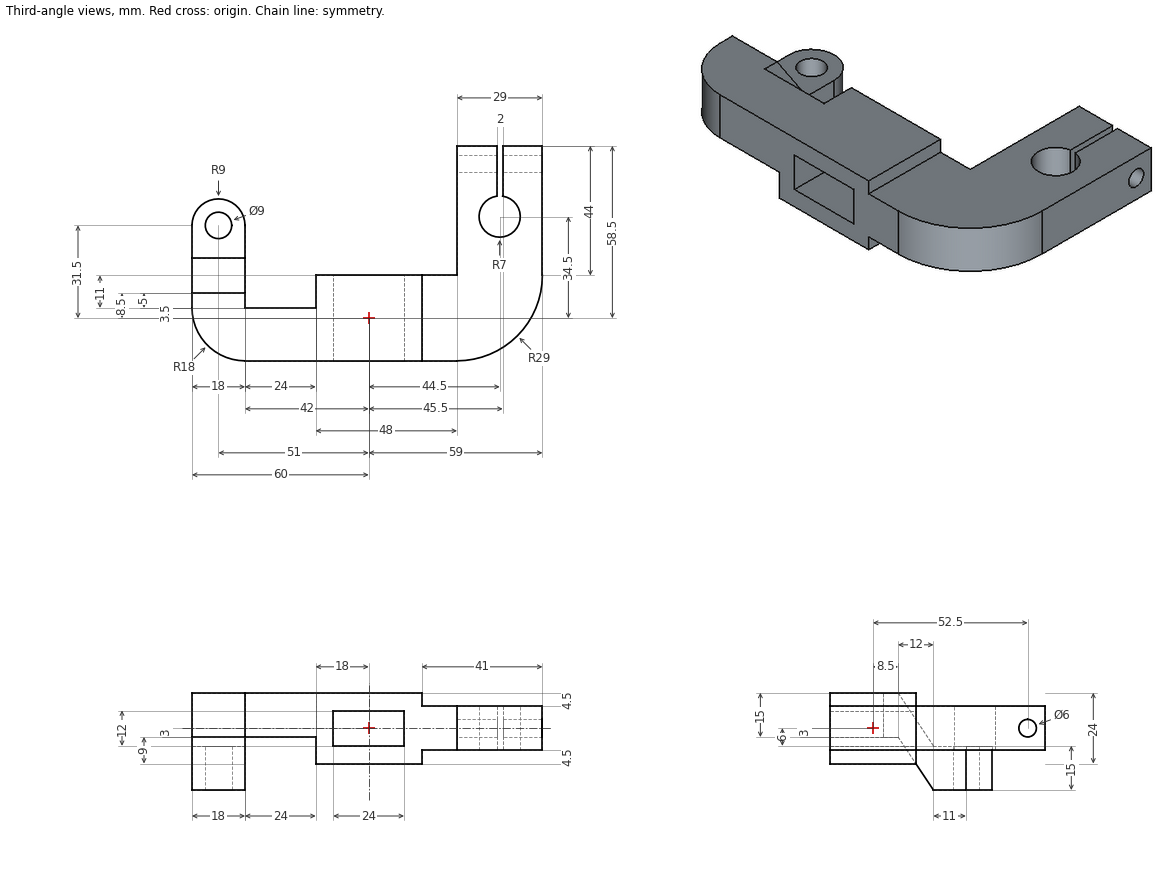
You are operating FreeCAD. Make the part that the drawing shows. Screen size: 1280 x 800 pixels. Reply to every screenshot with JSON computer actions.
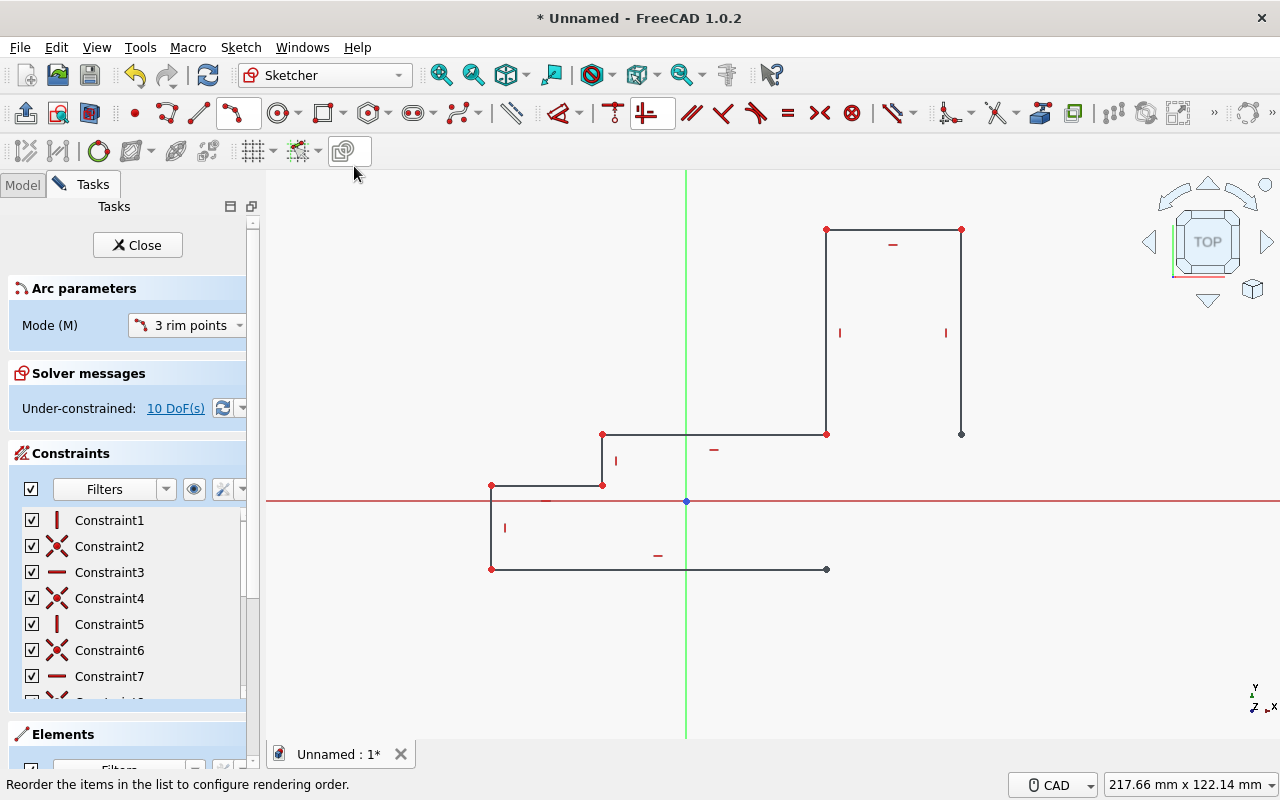
{"action": "left_click", "coordinate": [826, 570]}
{"action": "left_click", "coordinate": [961, 435]}
{"action": "left_click", "coordinate": [921, 529]}
{"action": "key", "text": "Escape"}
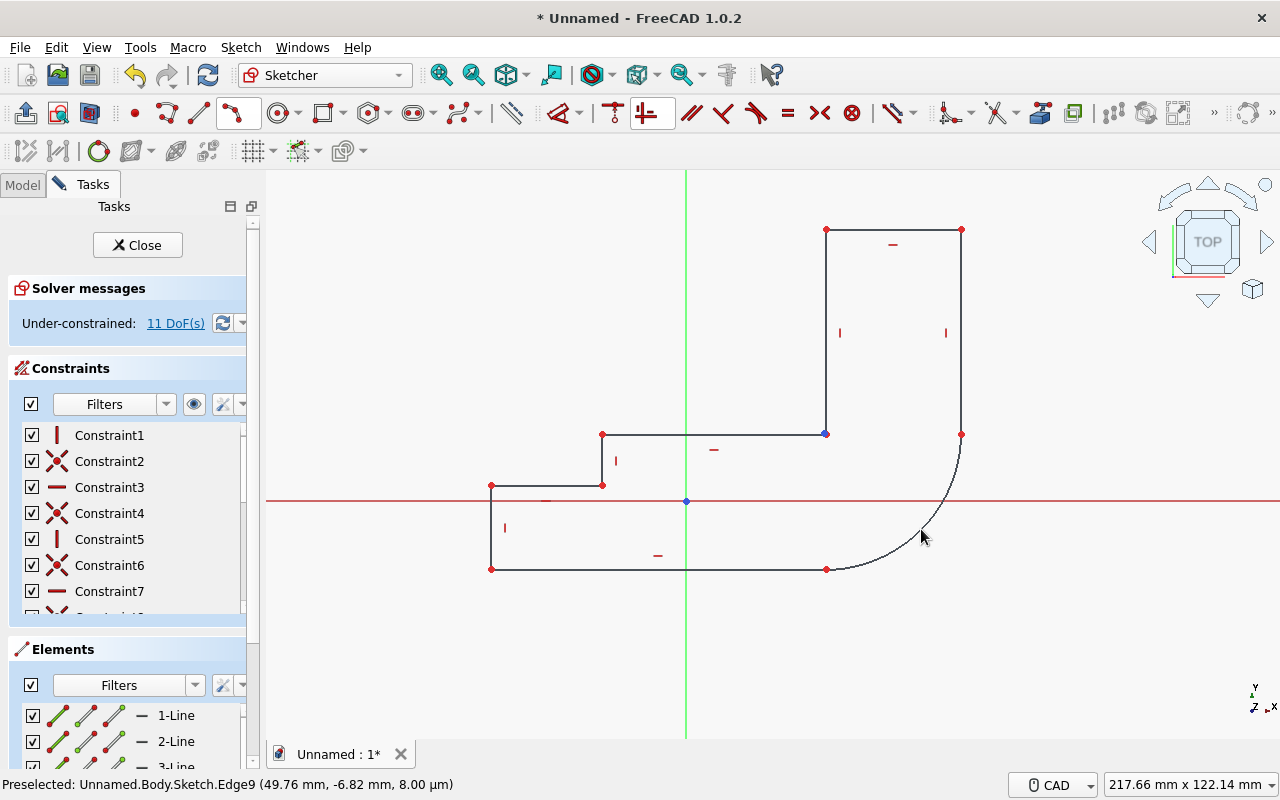
{"action": "left_click", "coordinate": [961, 373]}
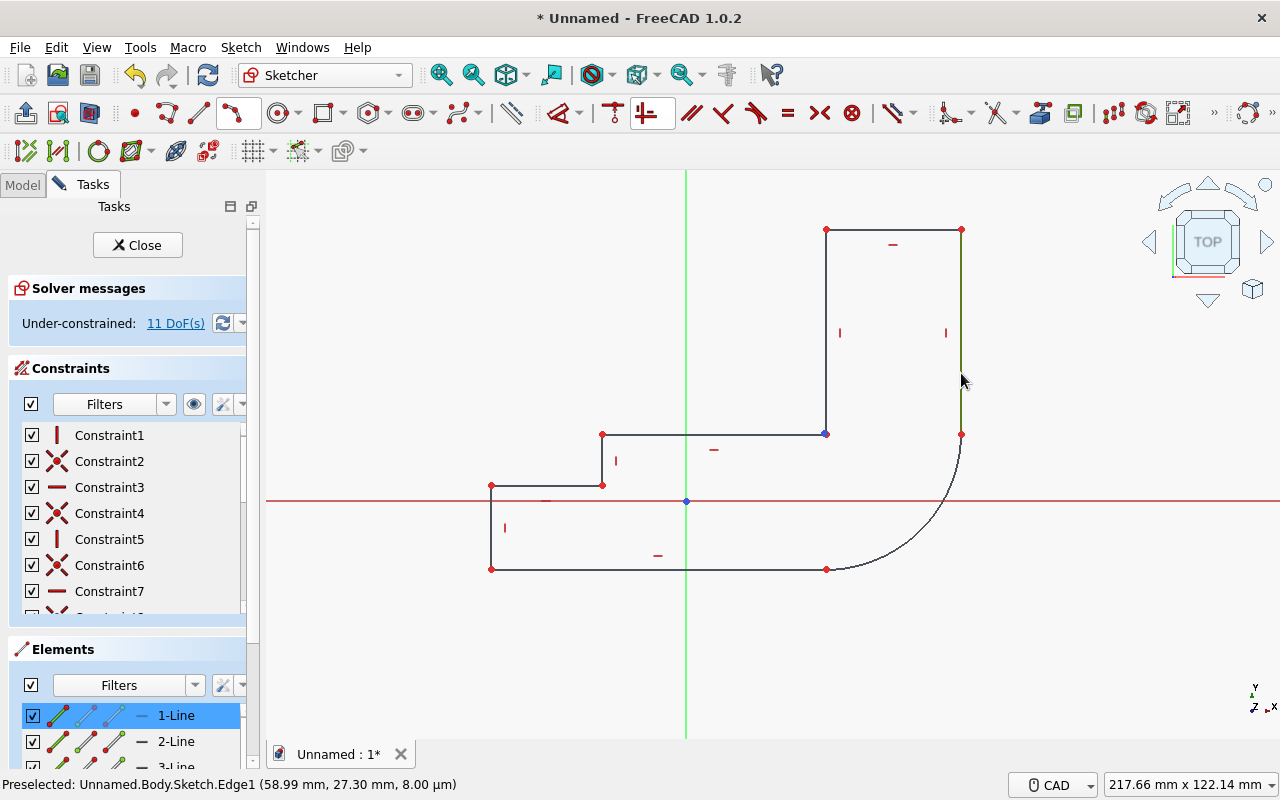
{"action": "left_click", "coordinate": [887, 555]}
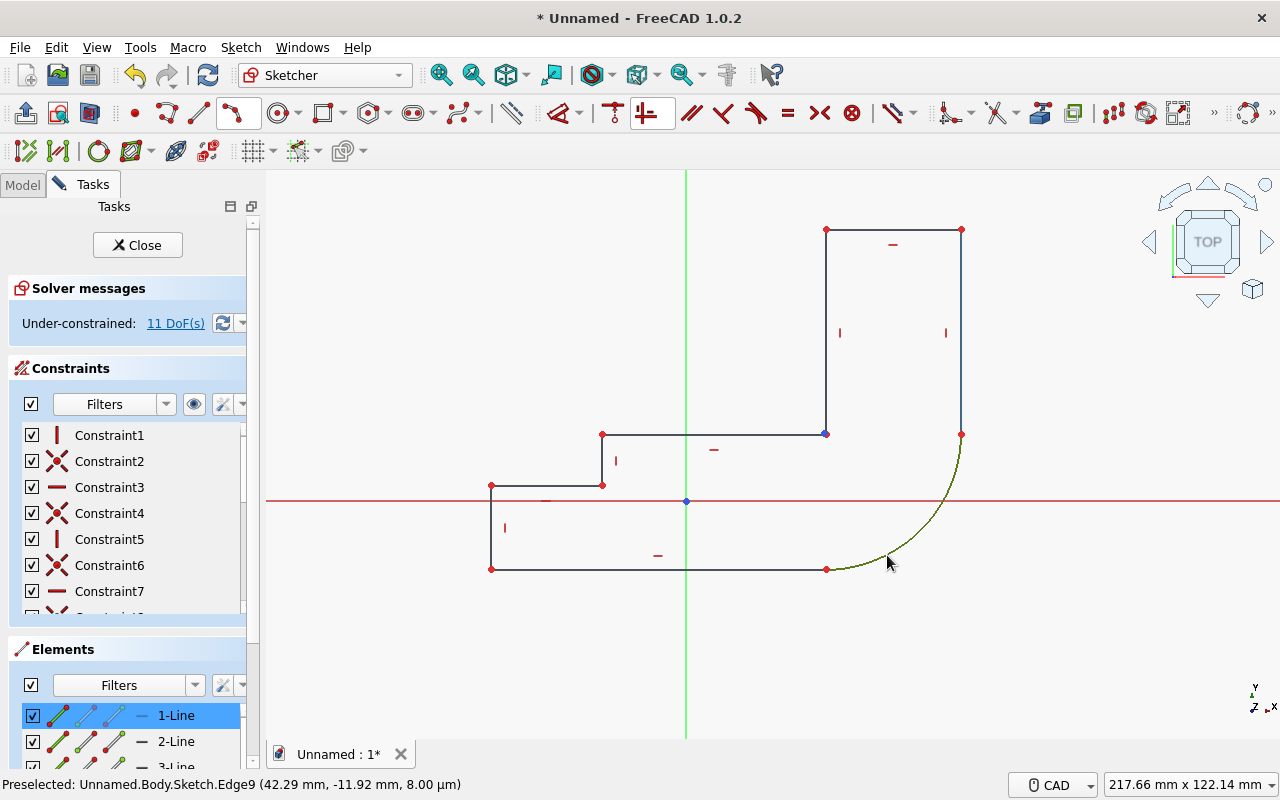
{"action": "left_click", "coordinate": [756, 114]}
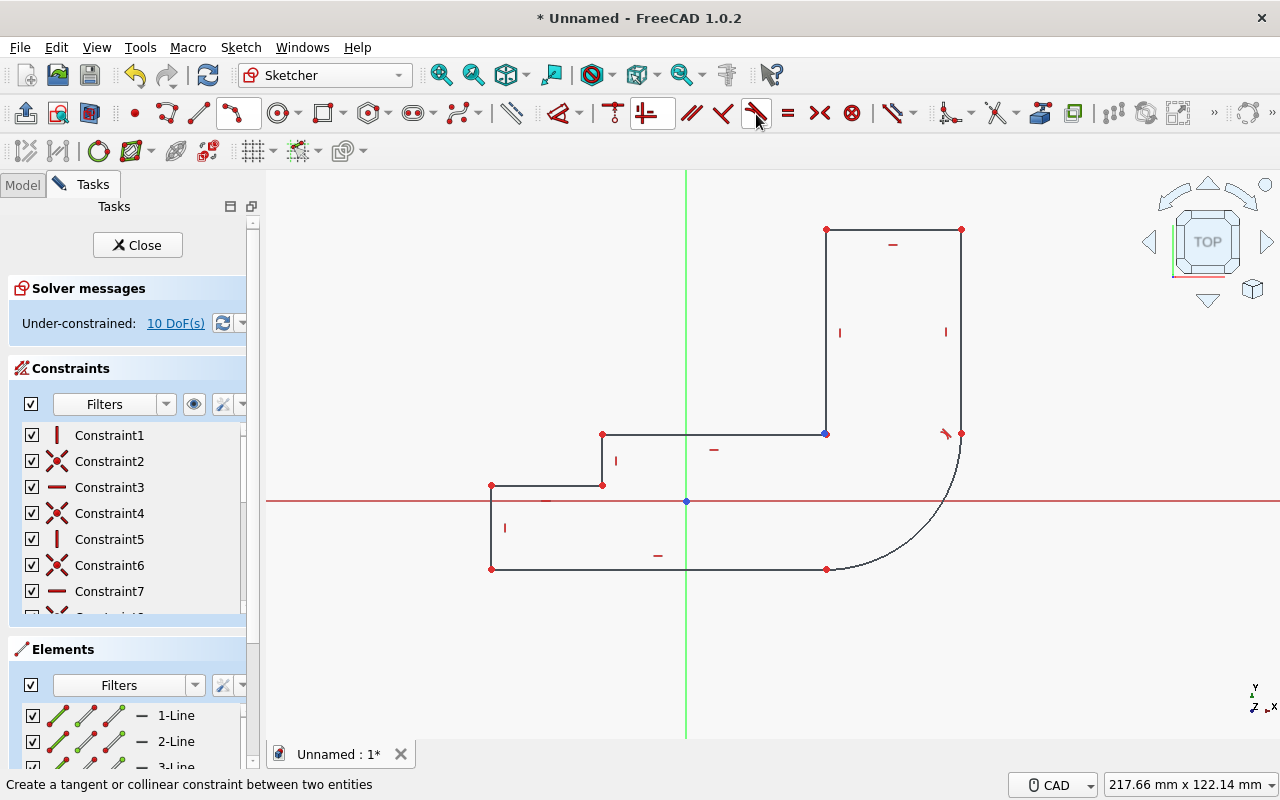
{"action": "left_click", "coordinate": [592, 570]}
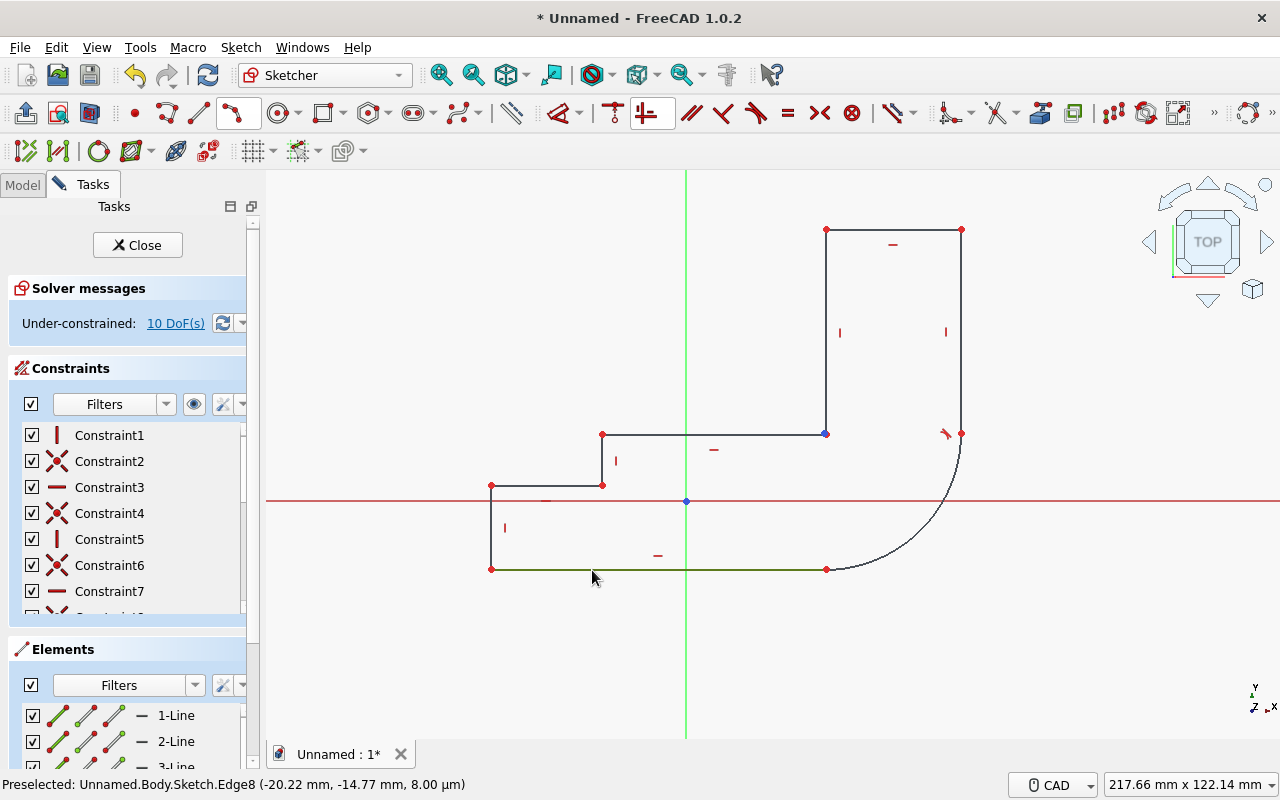
{"action": "left_click", "coordinate": [887, 555]}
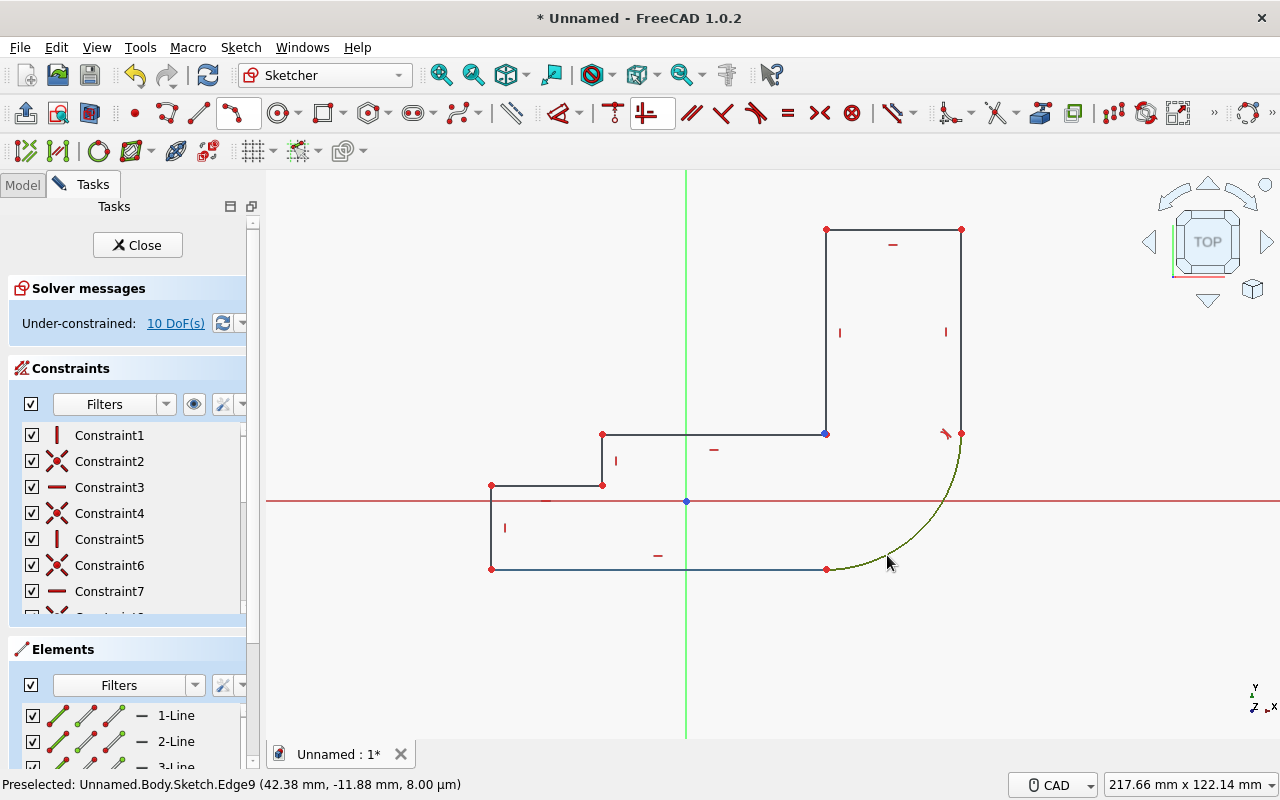
{"action": "left_click", "coordinate": [756, 114]}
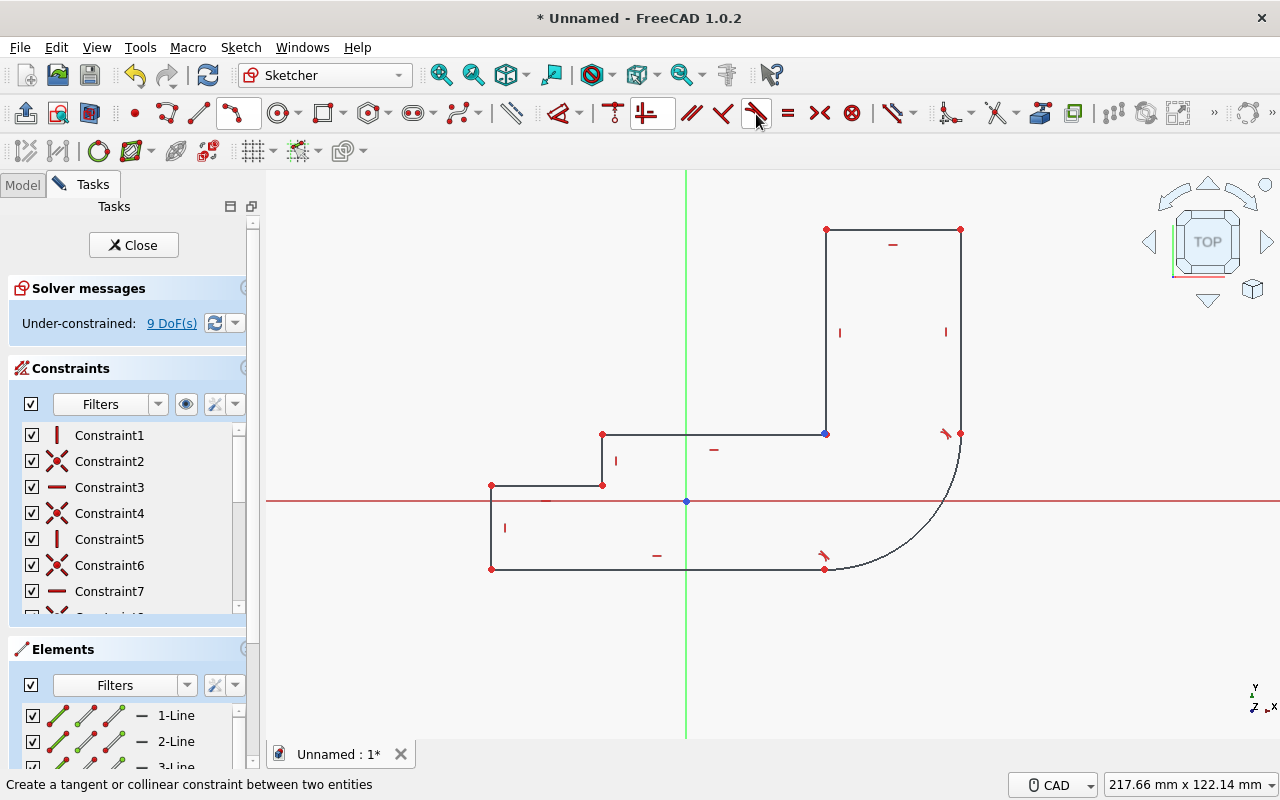
{"action": "left_click", "coordinate": [886, 555]}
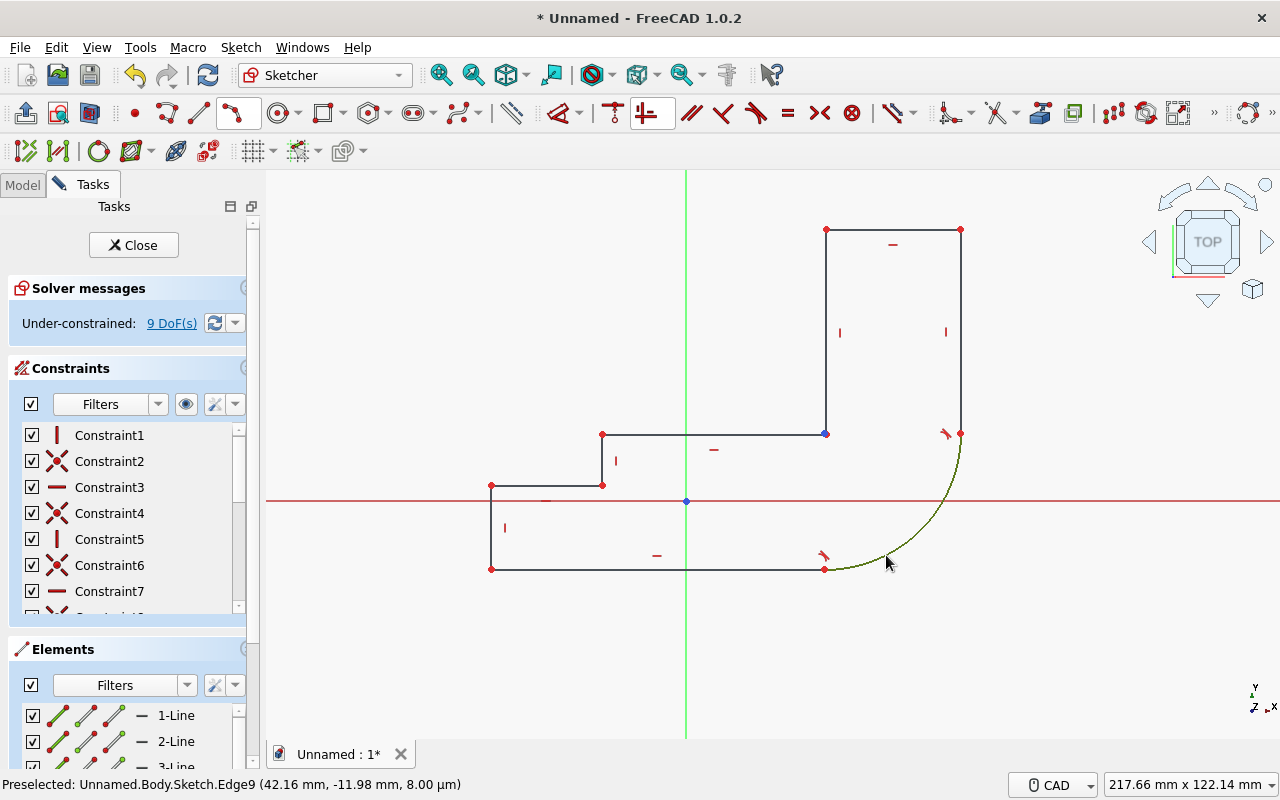
{"action": "left_click", "coordinate": [582, 114]}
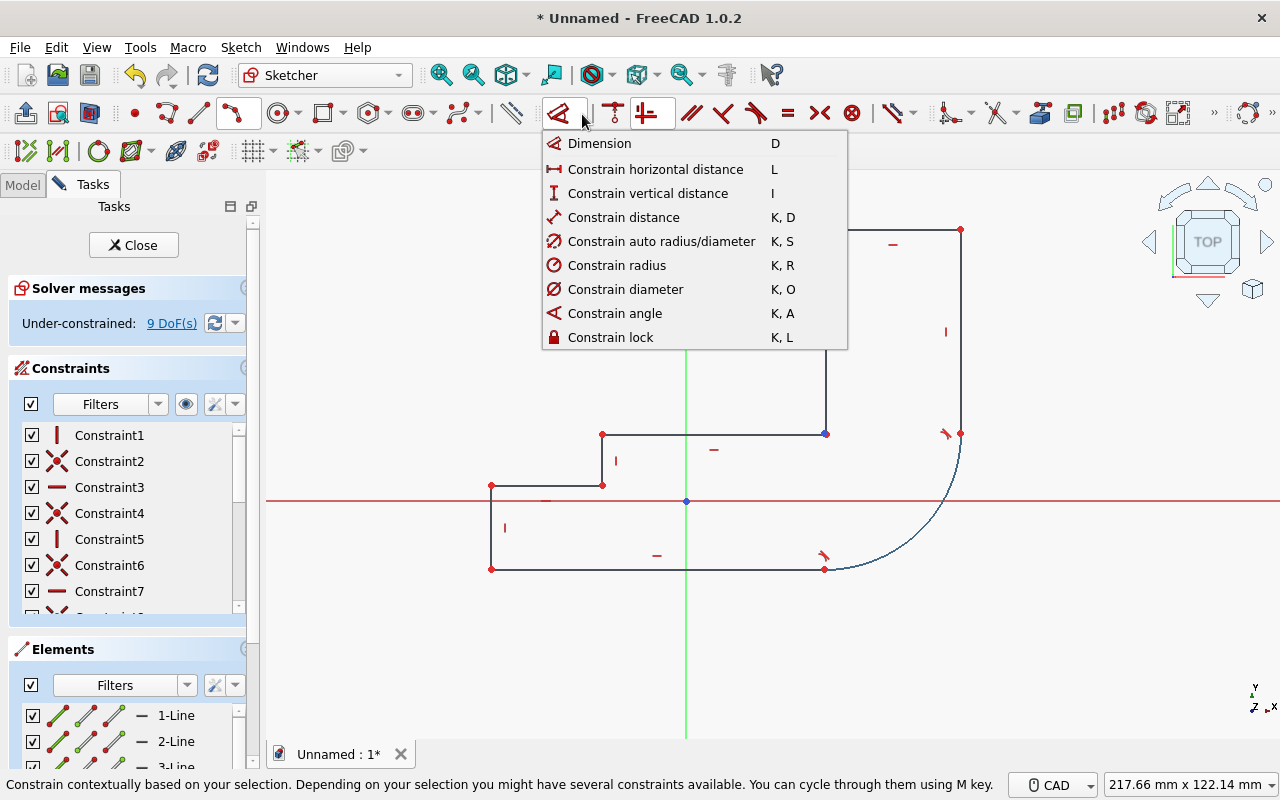
{"action": "left_click", "coordinate": [695, 265]}